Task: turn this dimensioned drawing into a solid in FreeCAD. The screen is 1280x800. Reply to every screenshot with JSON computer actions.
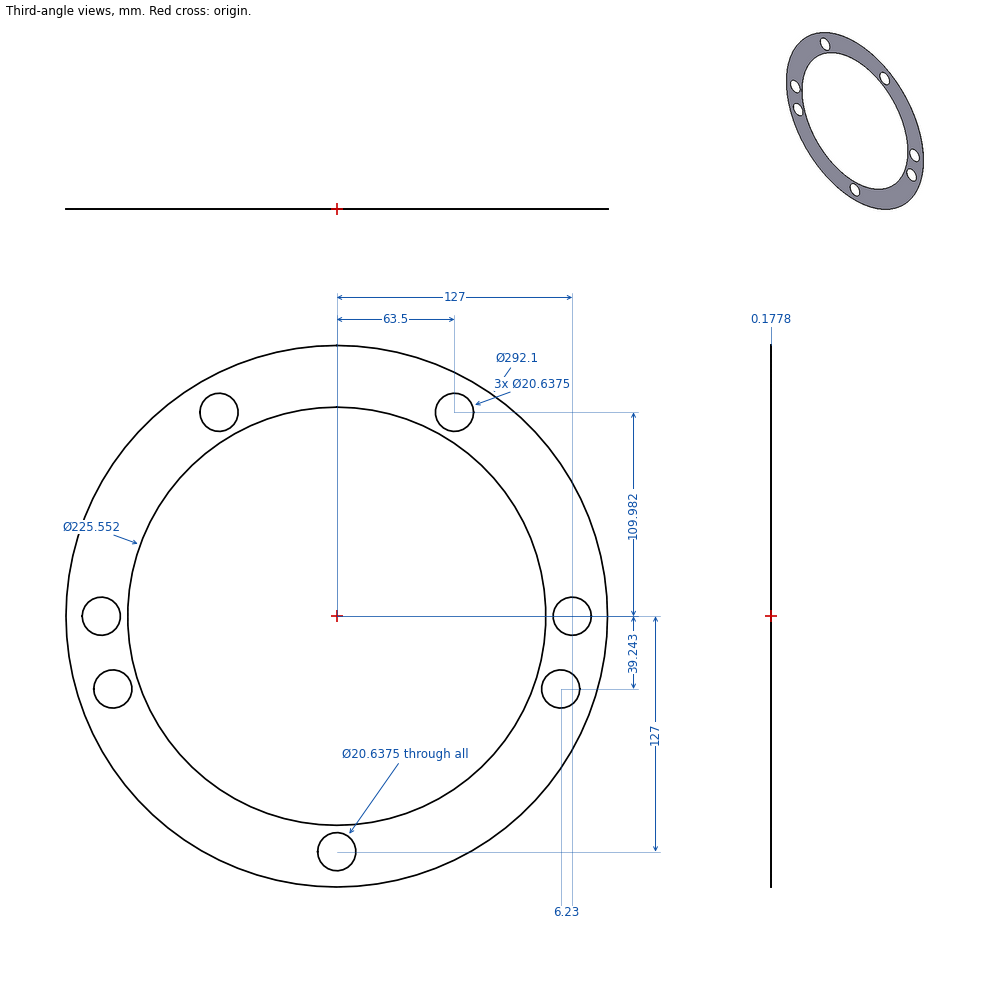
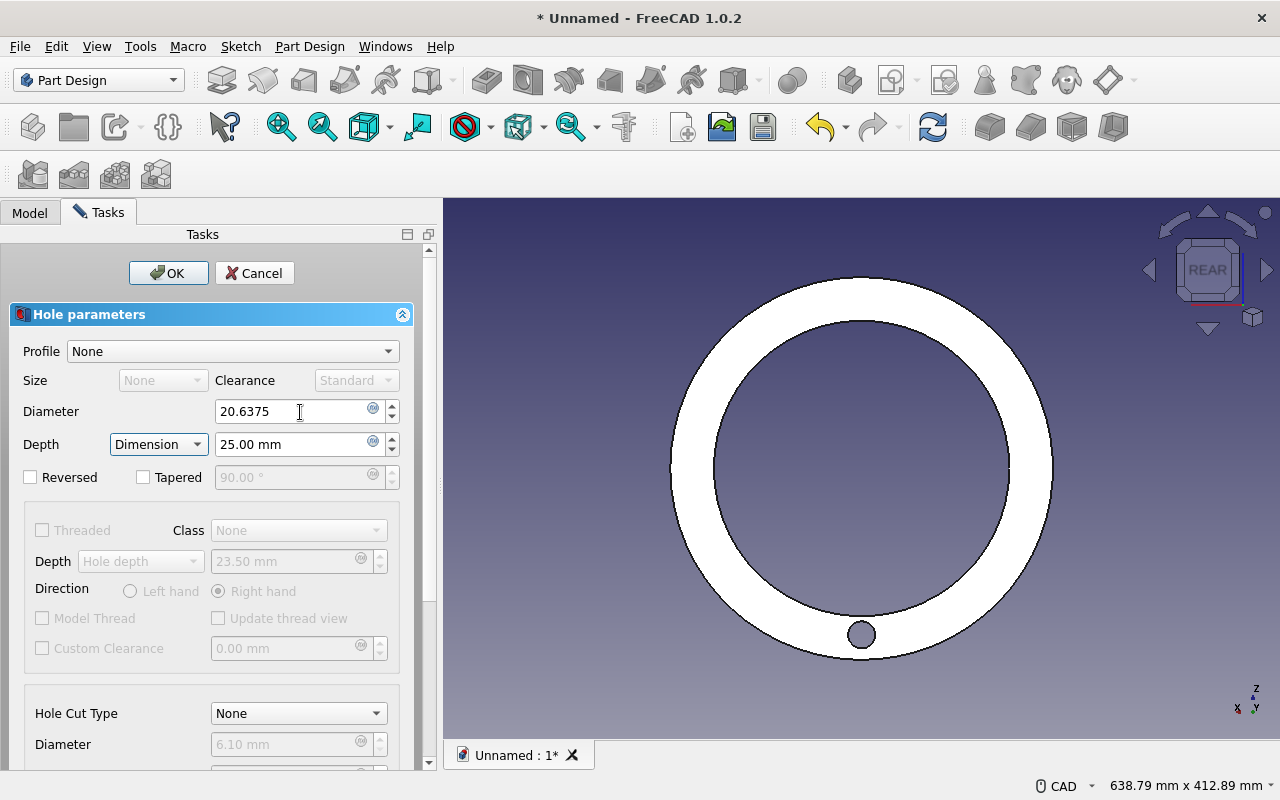
{"action": "left_click", "coordinate": [160, 444]}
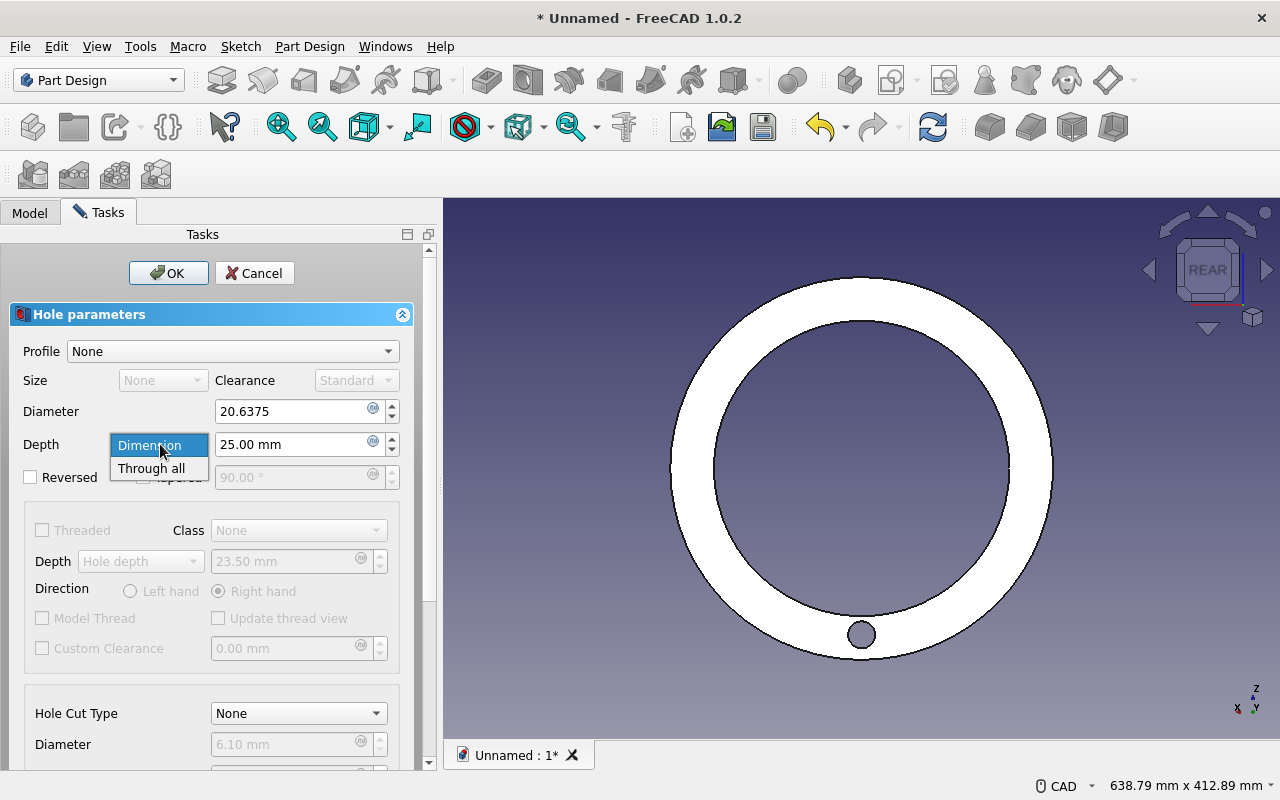
{"action": "left_click", "coordinate": [158, 468]}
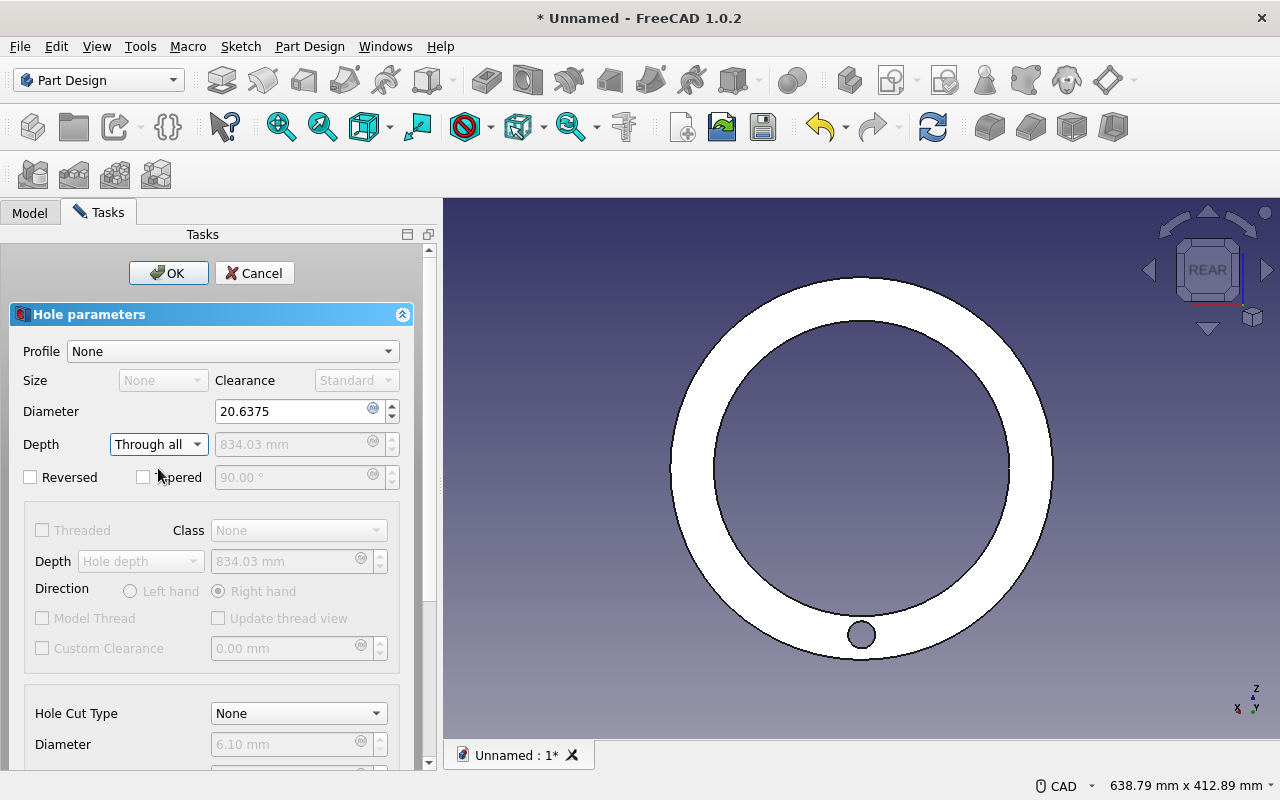
{"action": "left_click", "coordinate": [169, 273]}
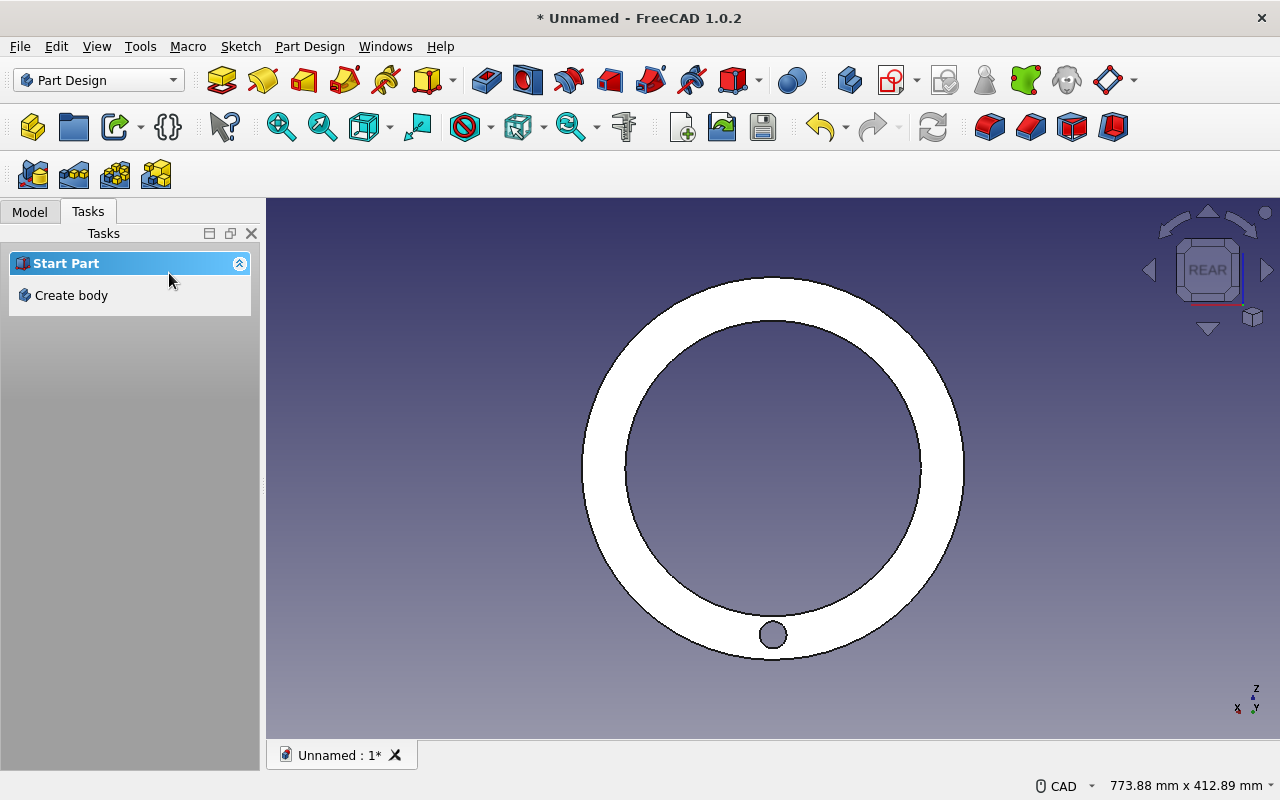
{"action": "left_click", "coordinate": [890, 80]}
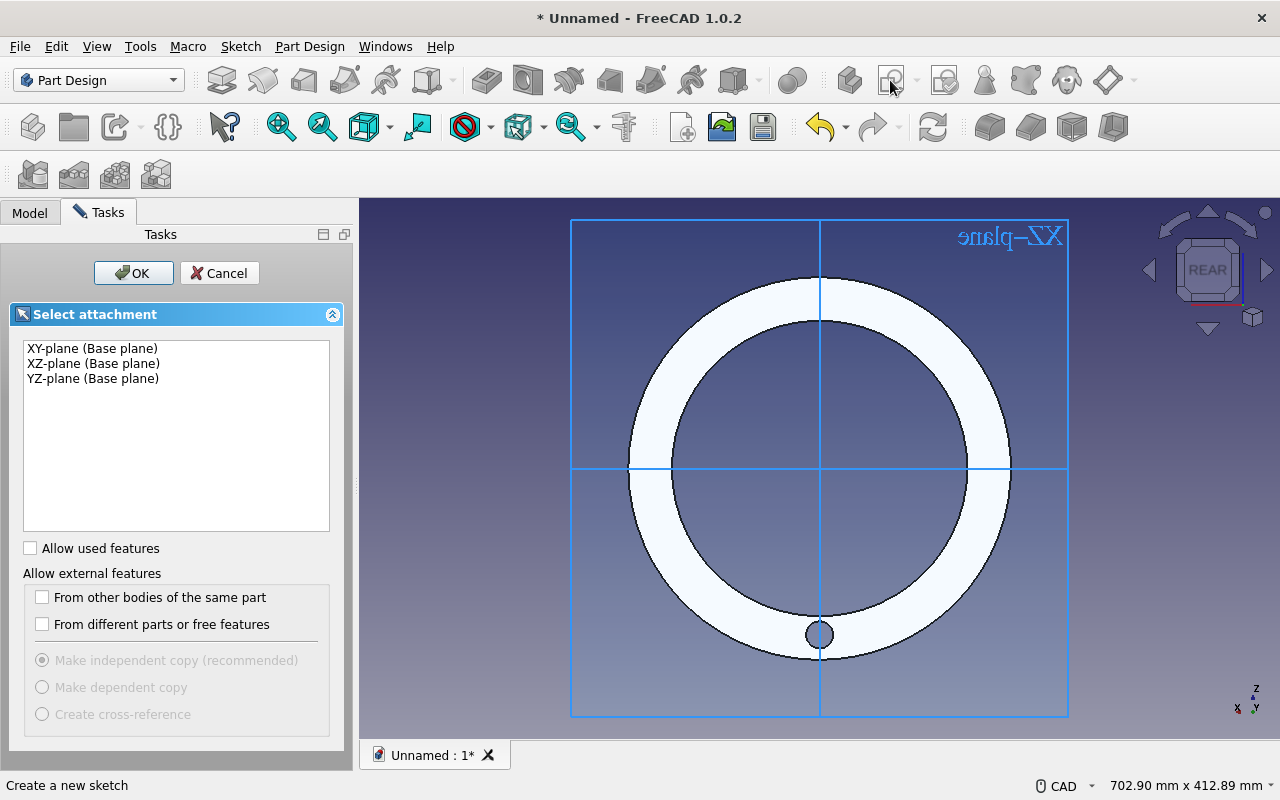
{"action": "left_click", "coordinate": [84, 364]}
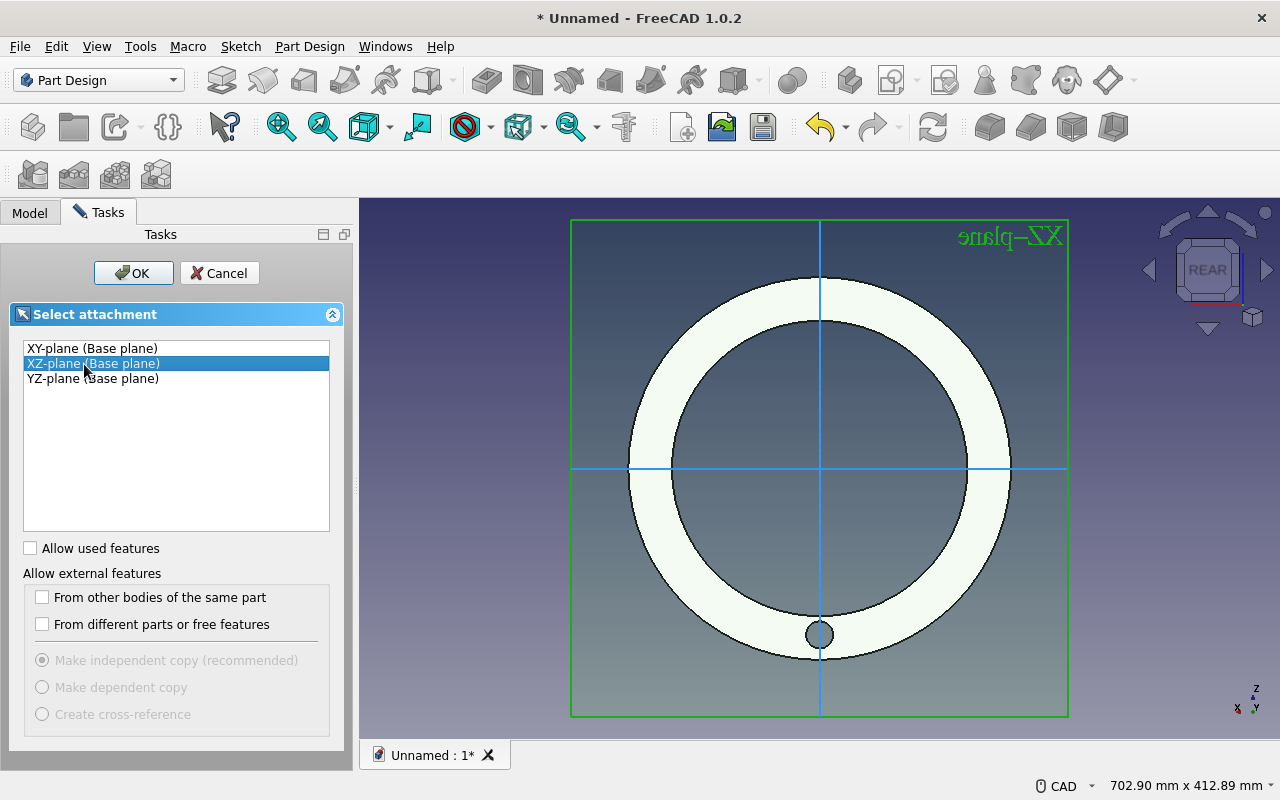
{"action": "left_click", "coordinate": [134, 273]}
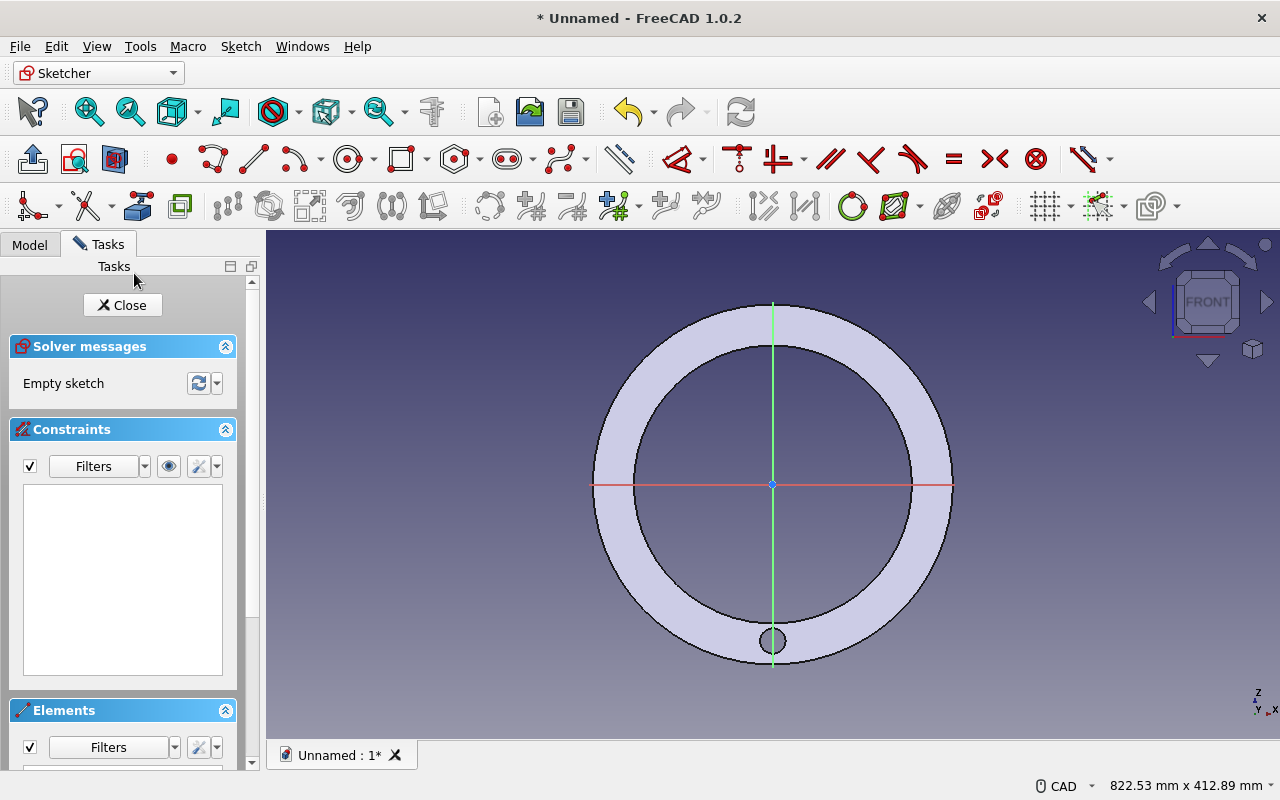
{"action": "scroll", "coordinate": [1115, 352], "scroll_direction": "up", "scroll_amount": 2}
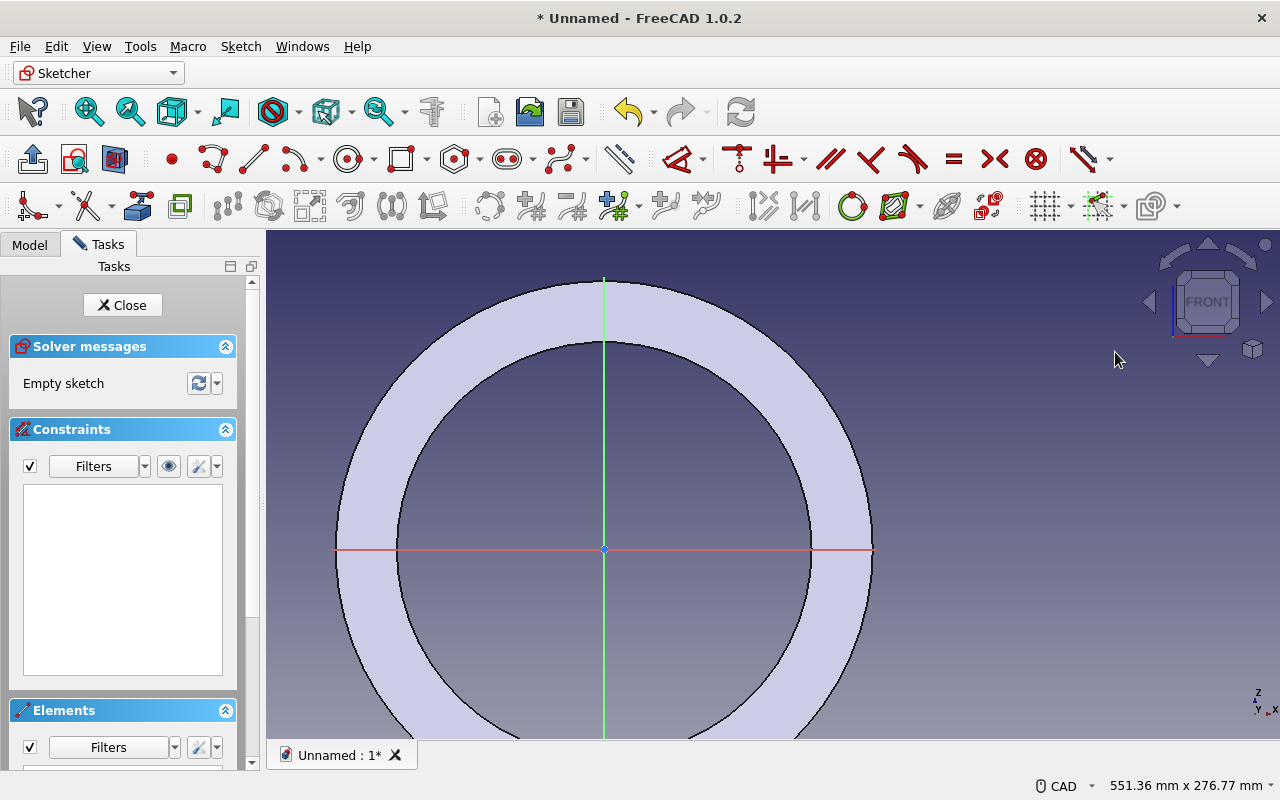
{"action": "key", "text": "g c"}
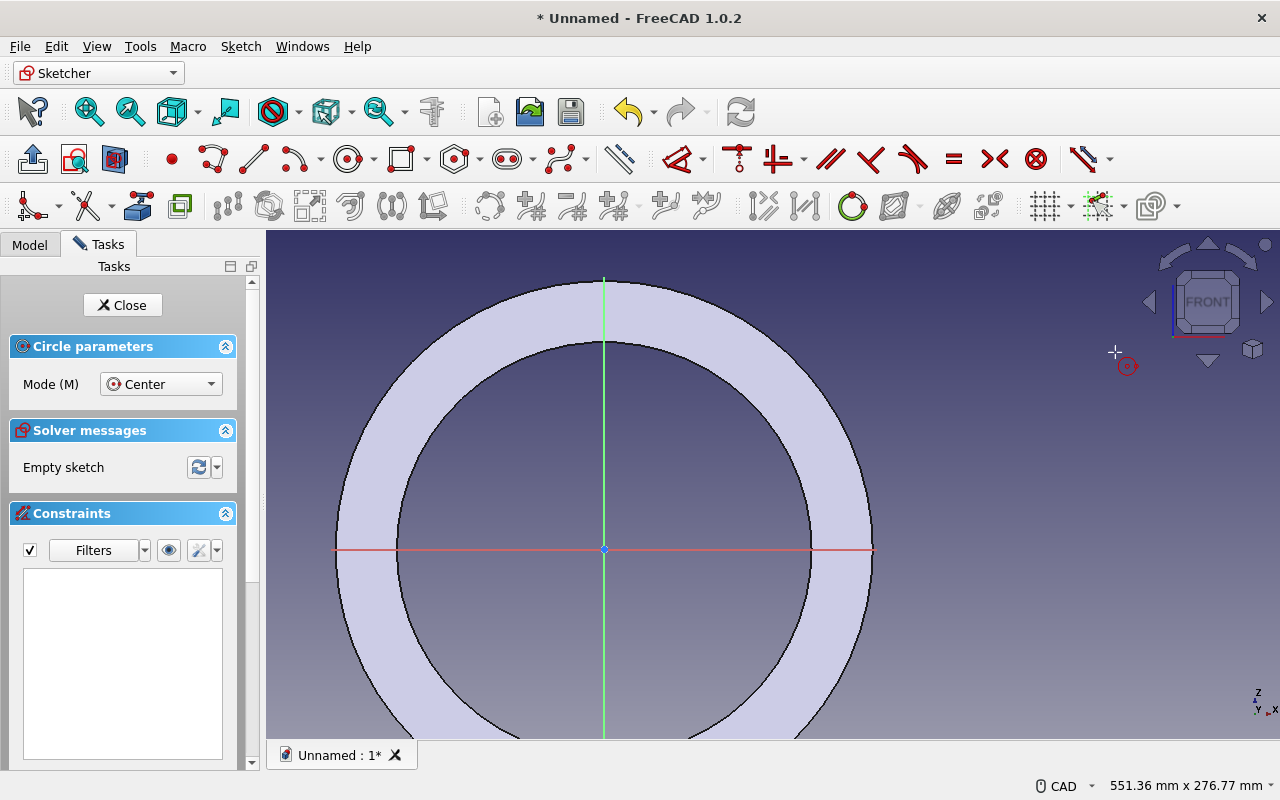
{"action": "left_click", "coordinate": [721, 347]}
{"action": "mouse_move", "coordinate": [734, 334]}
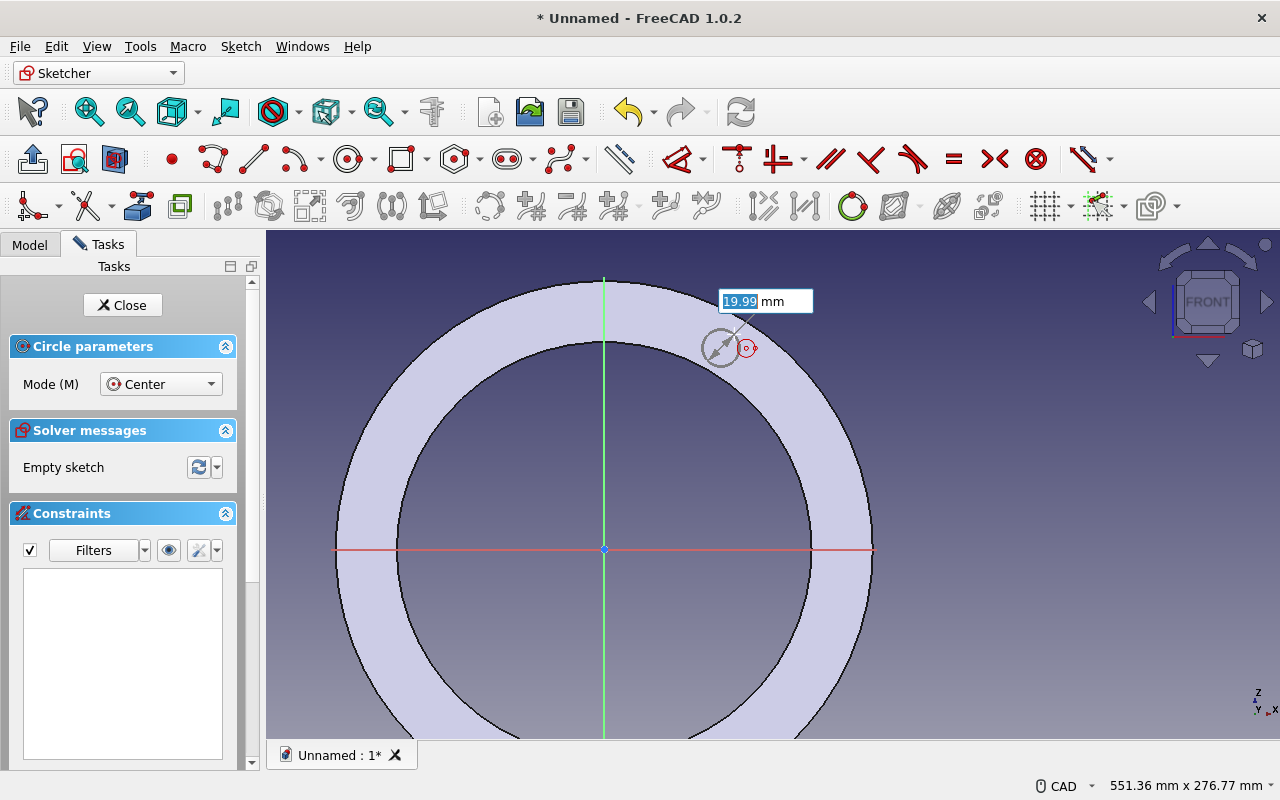
{"action": "type", "text": "20.6375"}
{"action": "key", "text": "Return"}